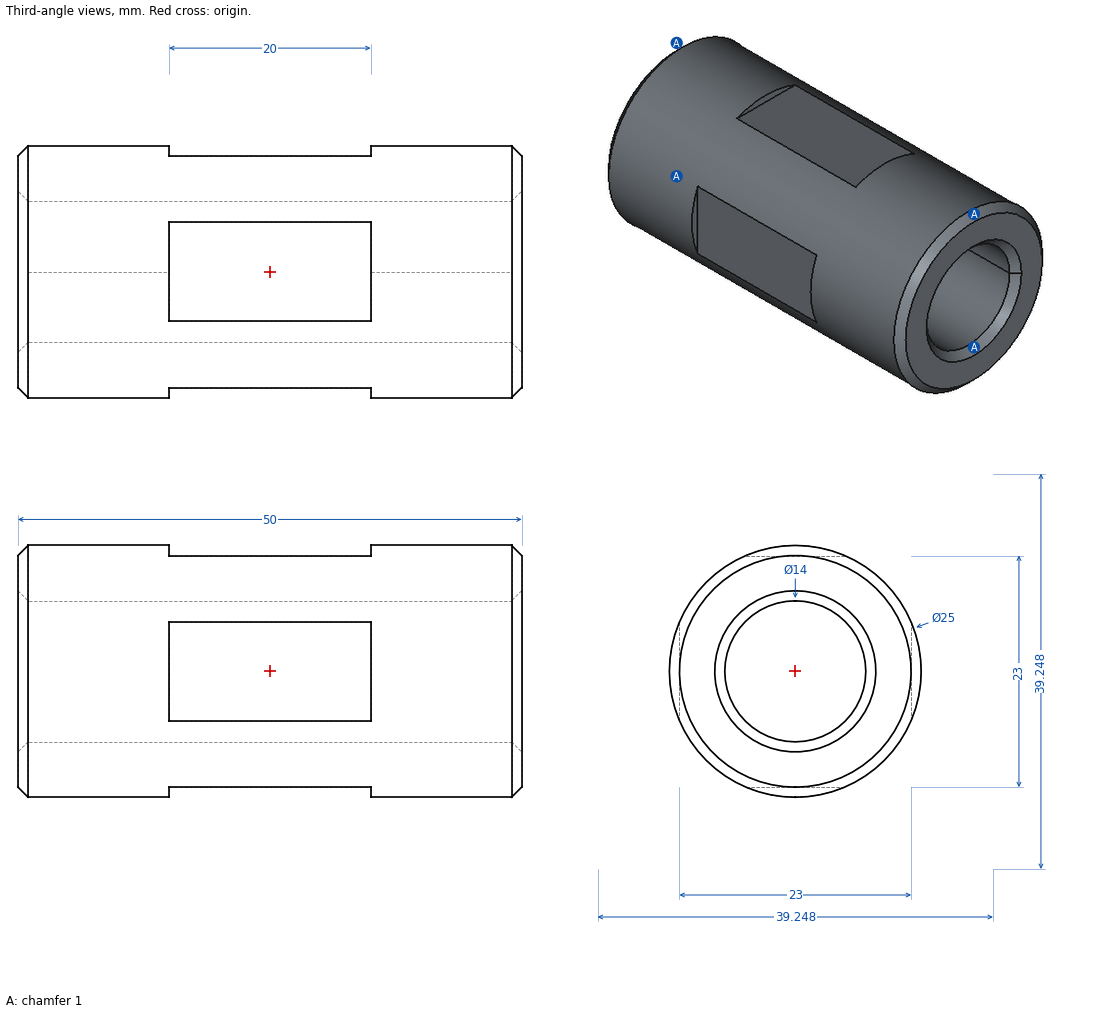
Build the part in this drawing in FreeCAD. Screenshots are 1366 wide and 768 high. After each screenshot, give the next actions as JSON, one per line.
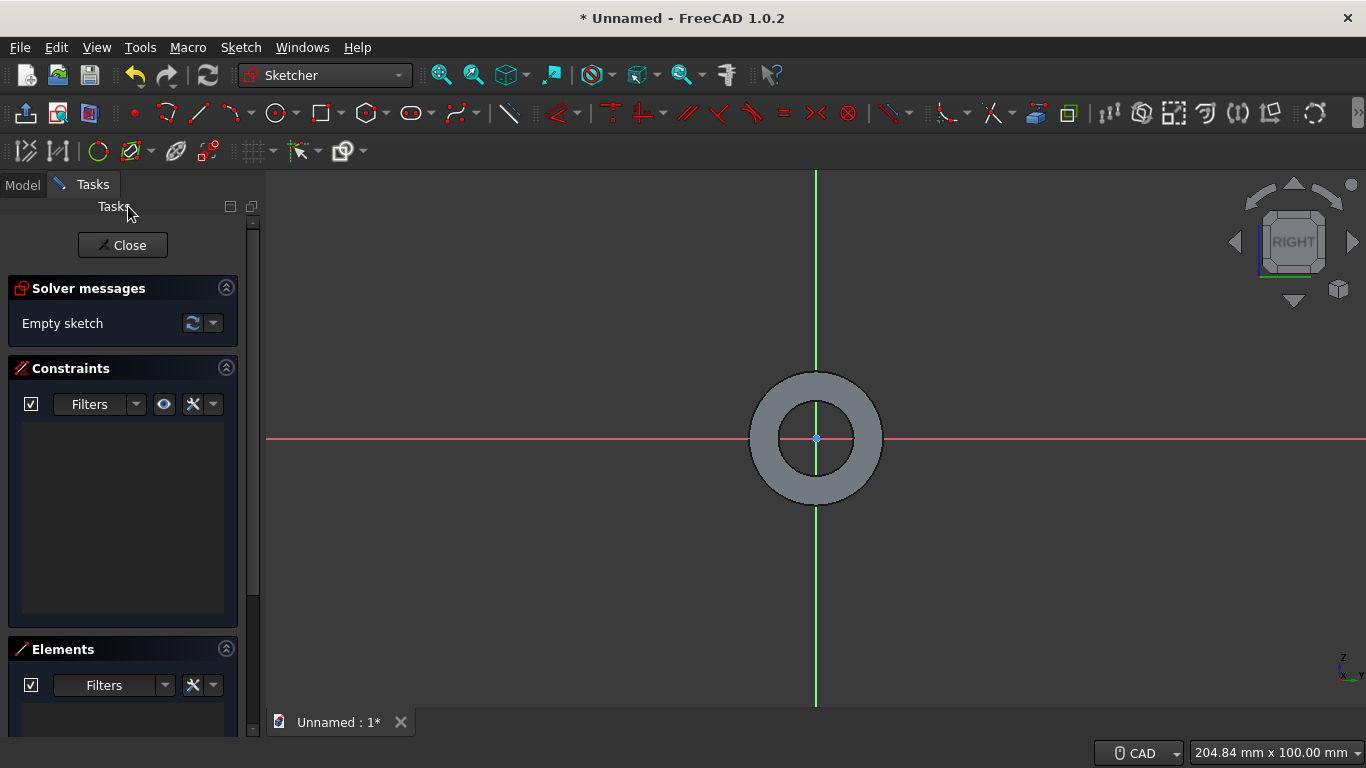
{"action": "left_click", "coordinate": [90, 114]}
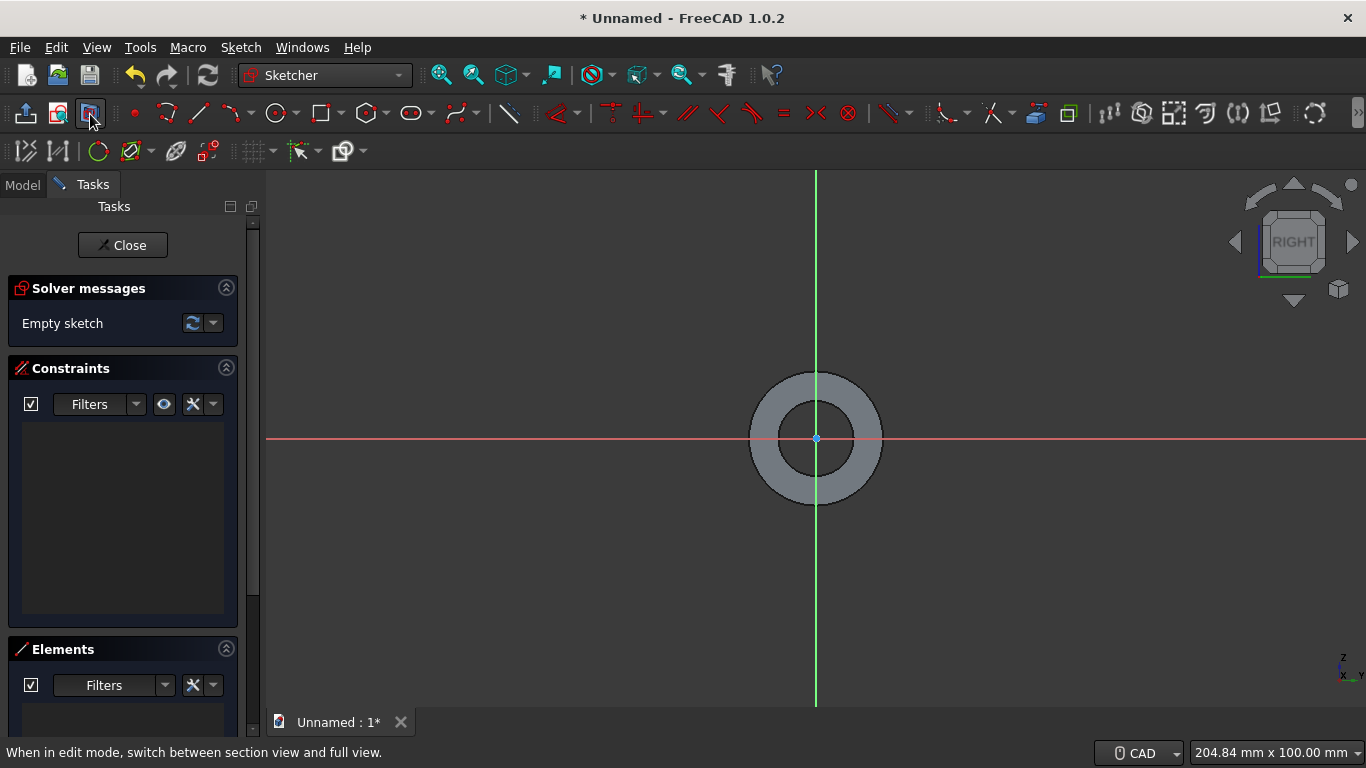
{"action": "scroll", "coordinate": [955, 439], "scroll_direction": "up", "scroll_amount": 2}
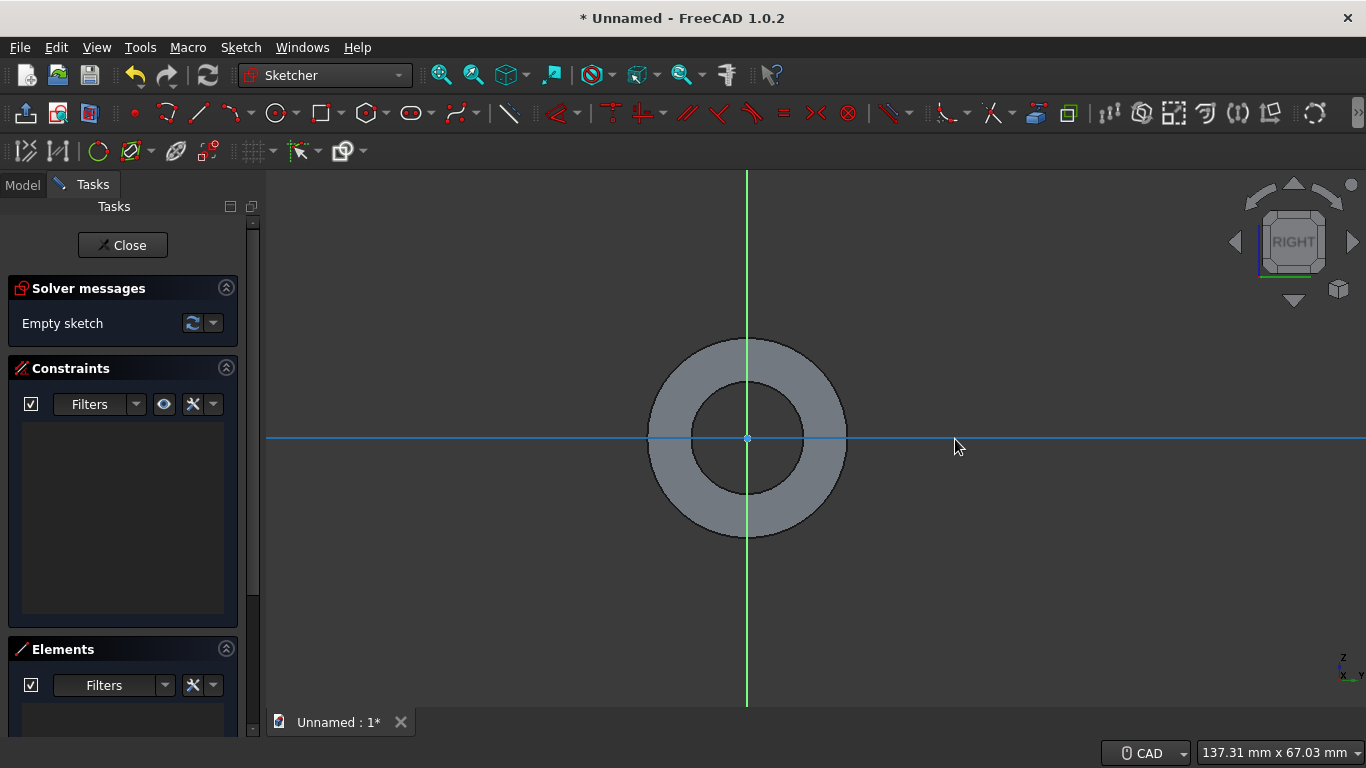
{"action": "left_click", "coordinate": [344, 114]}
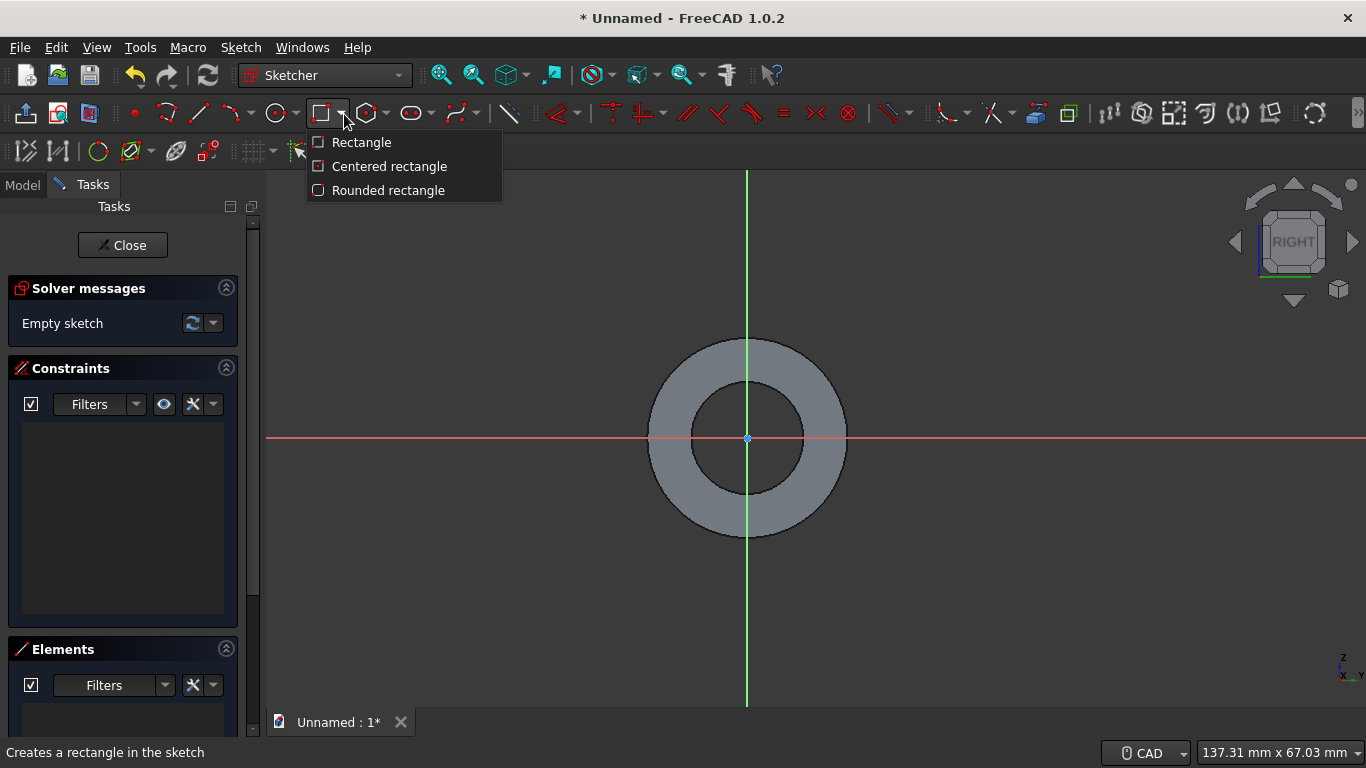
{"action": "left_click", "coordinate": [404, 166]}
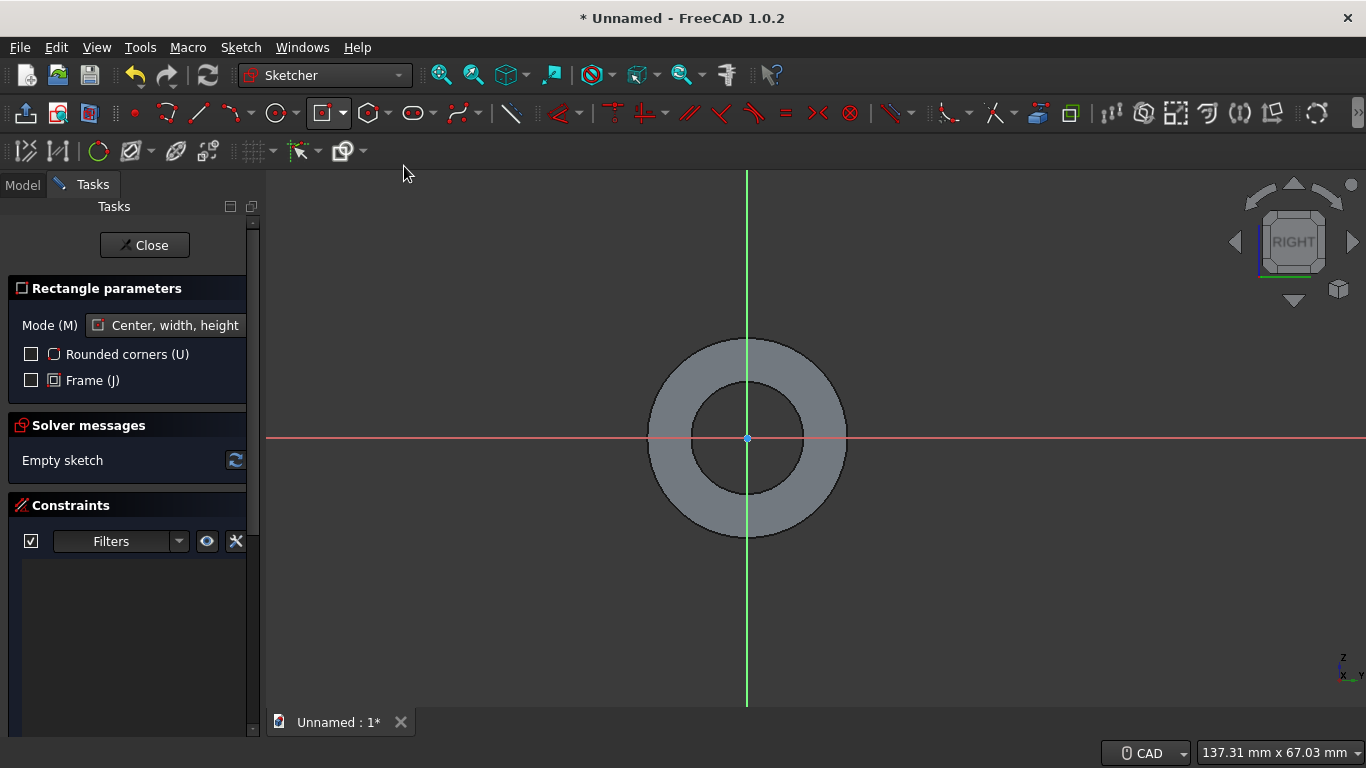
{"action": "left_click", "coordinate": [747, 438]}
{"action": "mouse_move", "coordinate": [905, 281]}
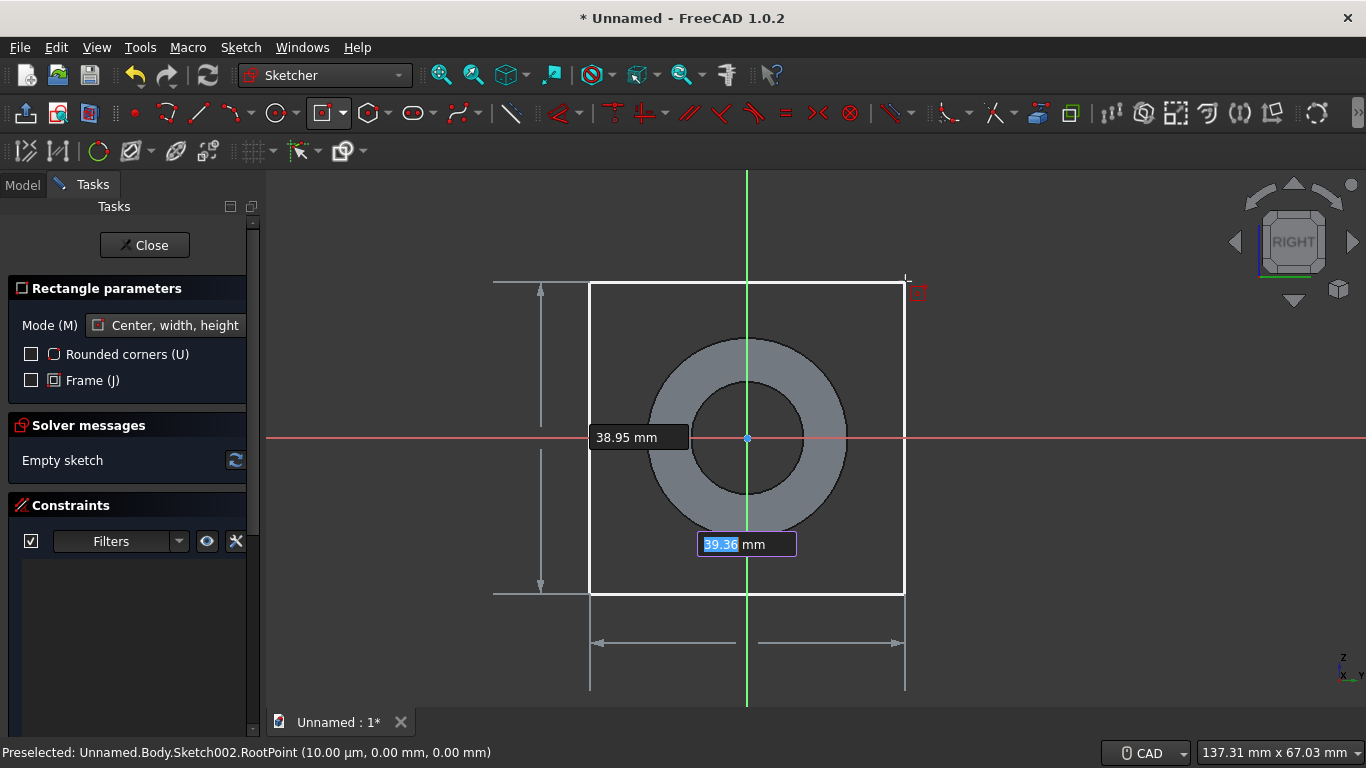
{"action": "type", "text": "39.248"}
{"action": "key", "text": "Tab"}
{"action": "type", "text": "39.248"}
{"action": "key", "text": "Return"}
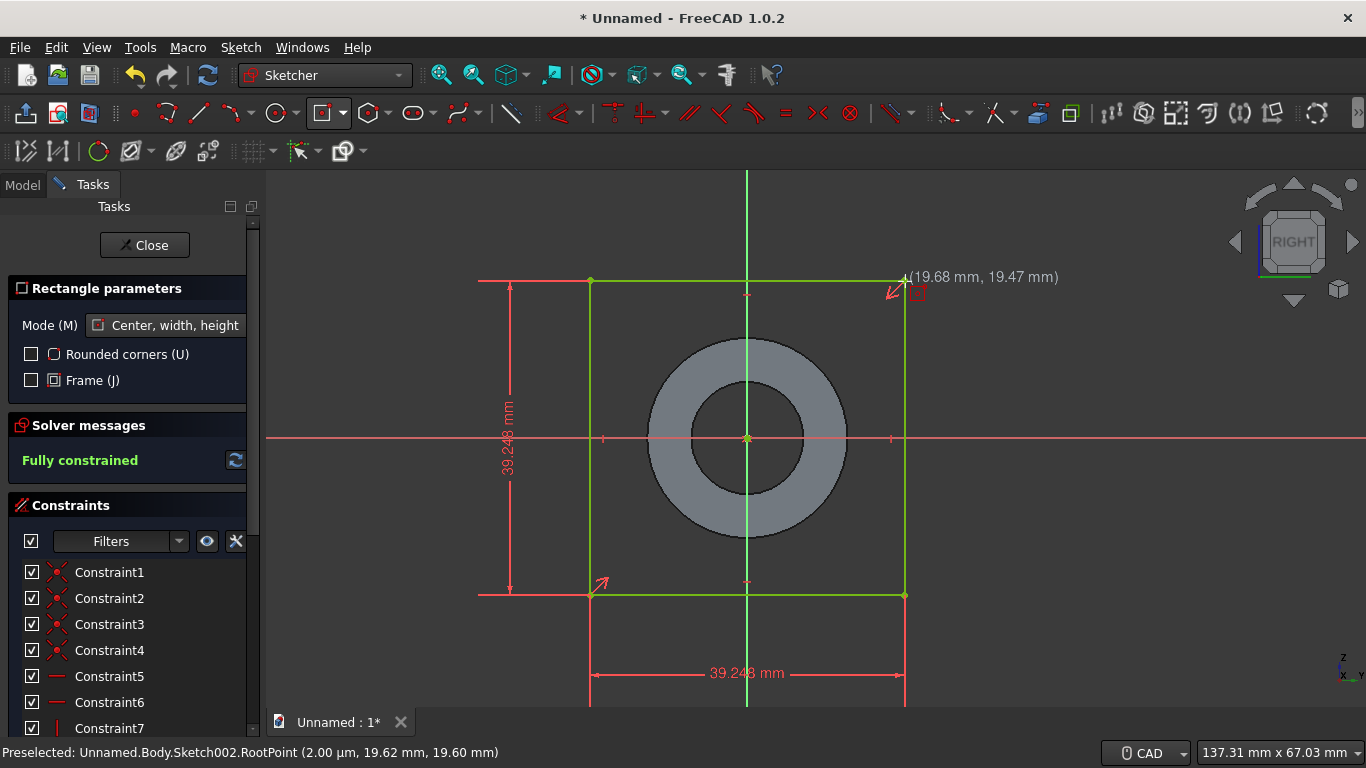
{"action": "left_click", "coordinate": [747, 438]}
{"action": "mouse_move", "coordinate": [839, 346]}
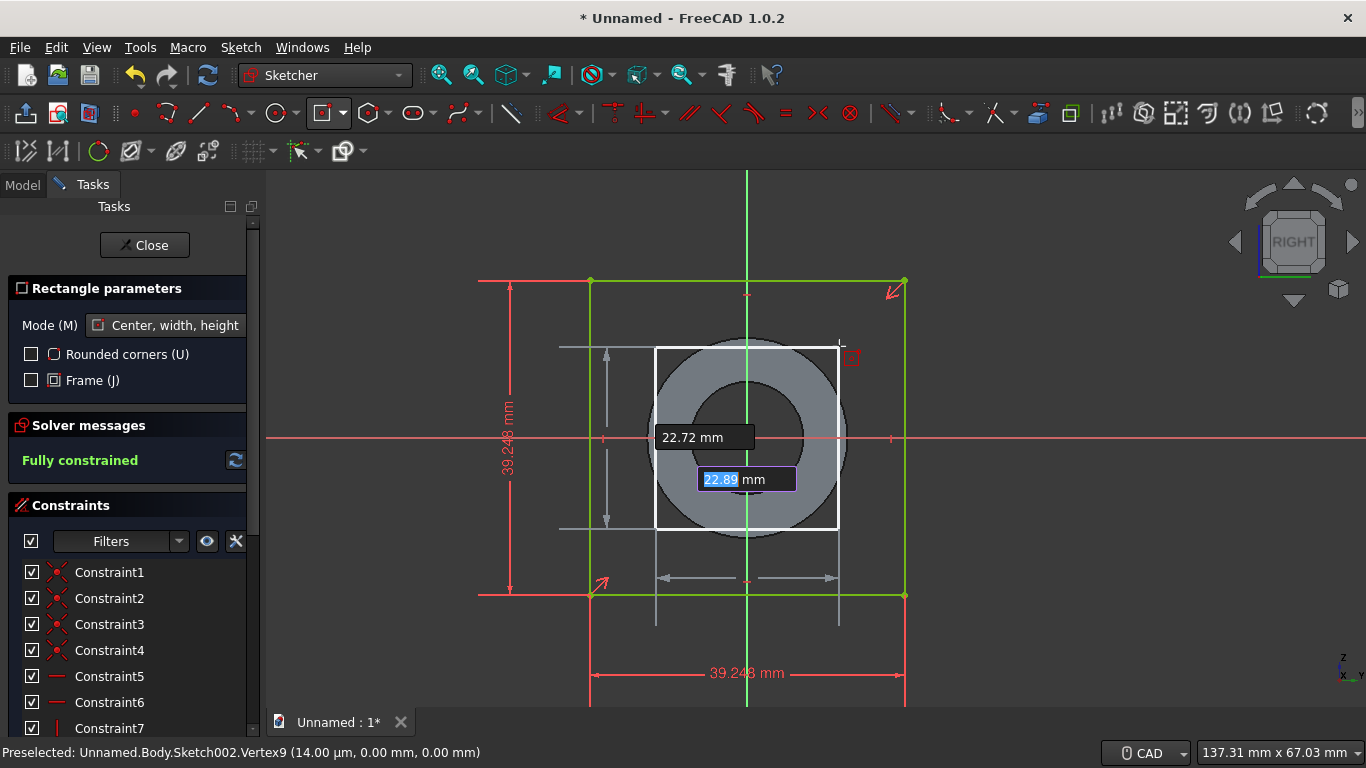
{"action": "type", "text": "23"}
{"action": "key", "text": "Tab"}
{"action": "type", "text": "23"}
{"action": "key", "text": "Return"}
{"action": "key", "text": "Escape"}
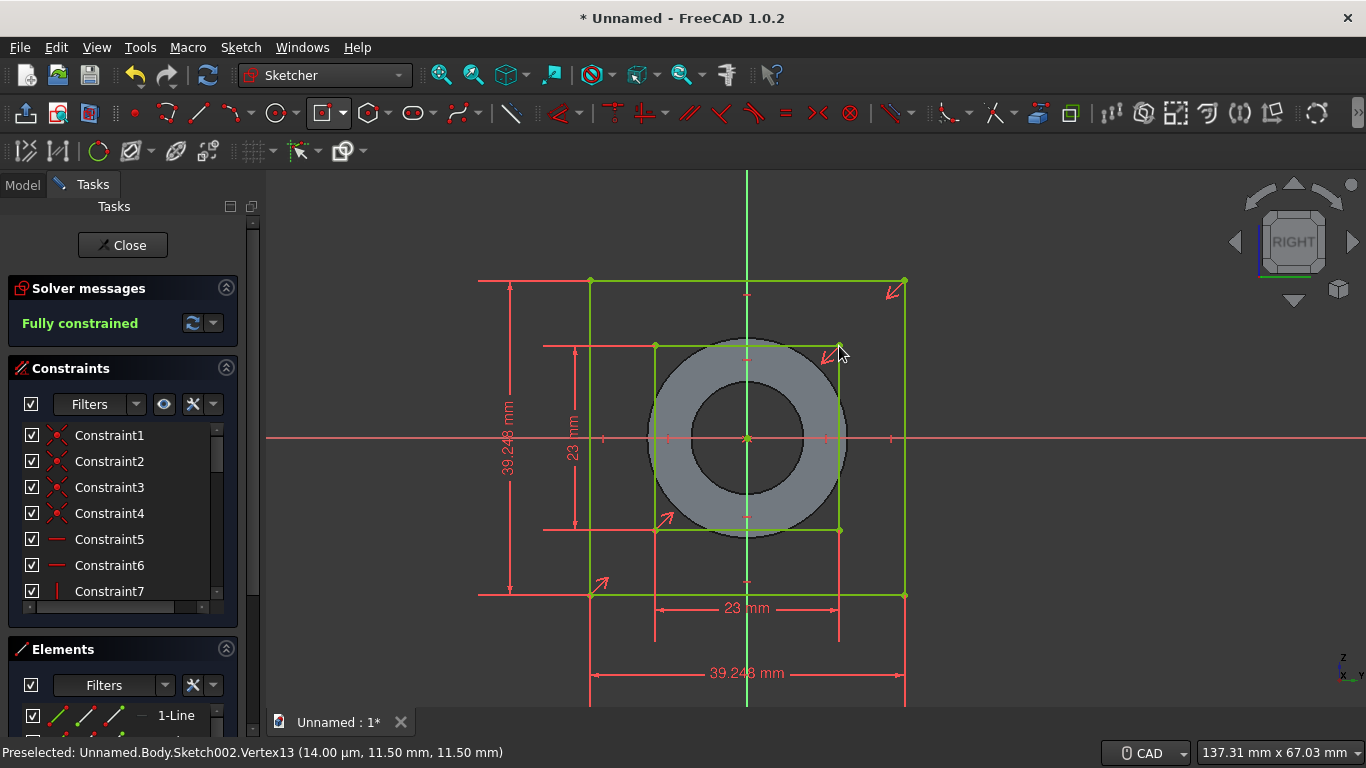
{"action": "left_click", "coordinate": [123, 245]}